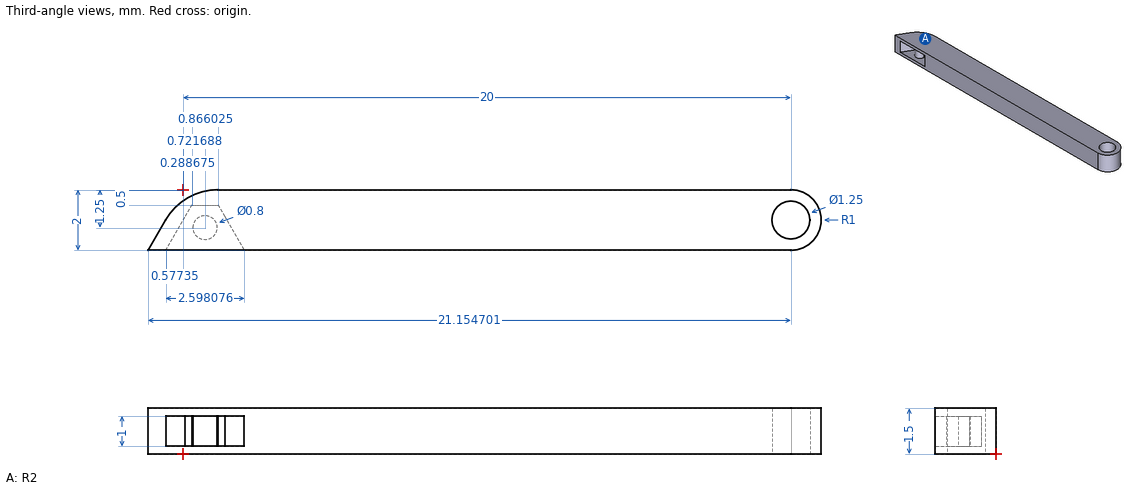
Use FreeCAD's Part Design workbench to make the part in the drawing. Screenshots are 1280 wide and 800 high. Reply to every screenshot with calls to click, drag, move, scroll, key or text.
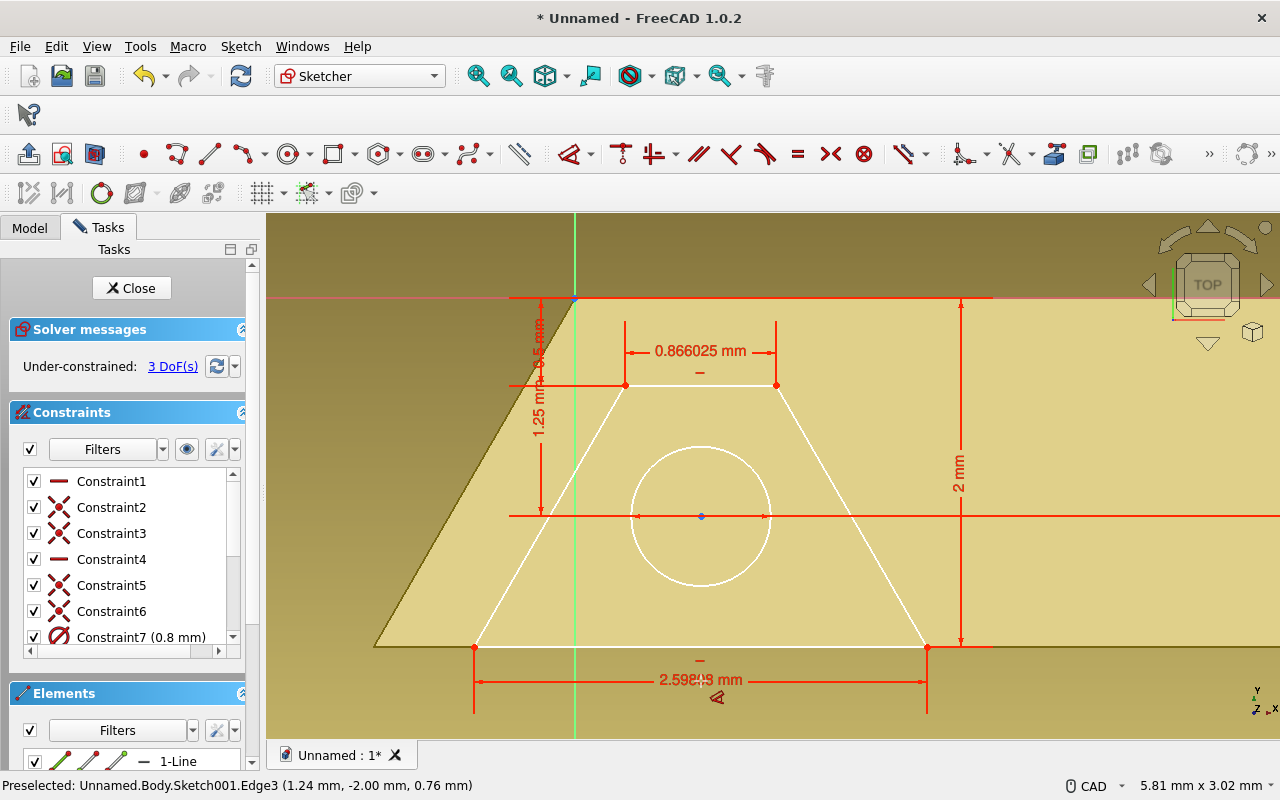
click(474, 647)
click(524, 681)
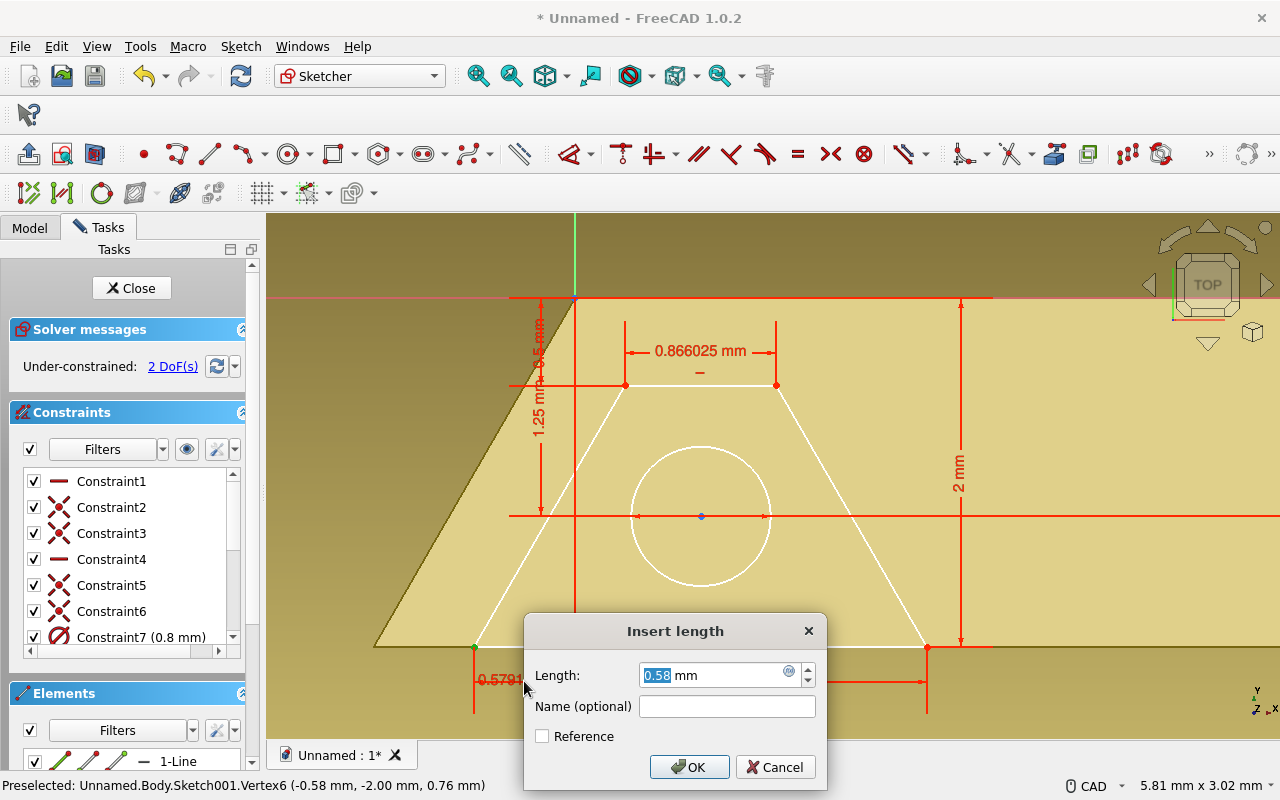
text(0.57735)
key(Return)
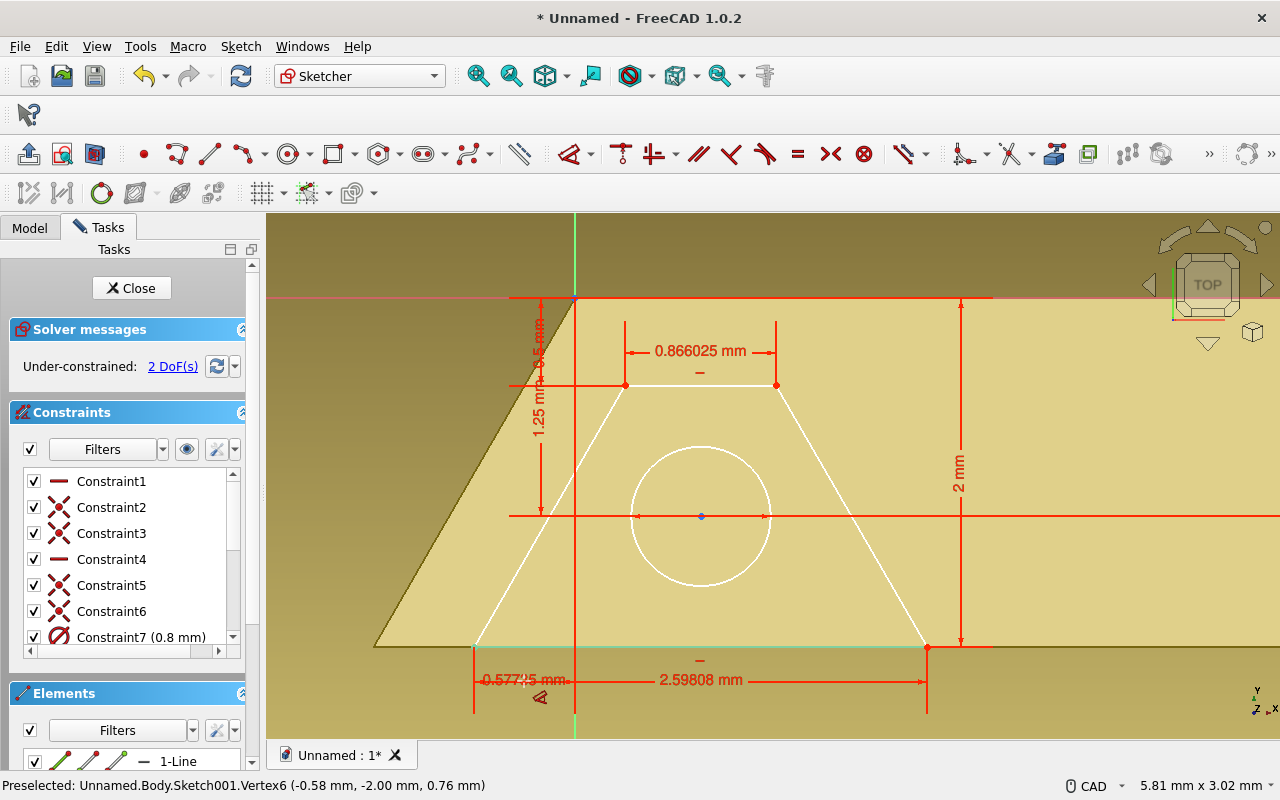
click(701, 516)
click(638, 264)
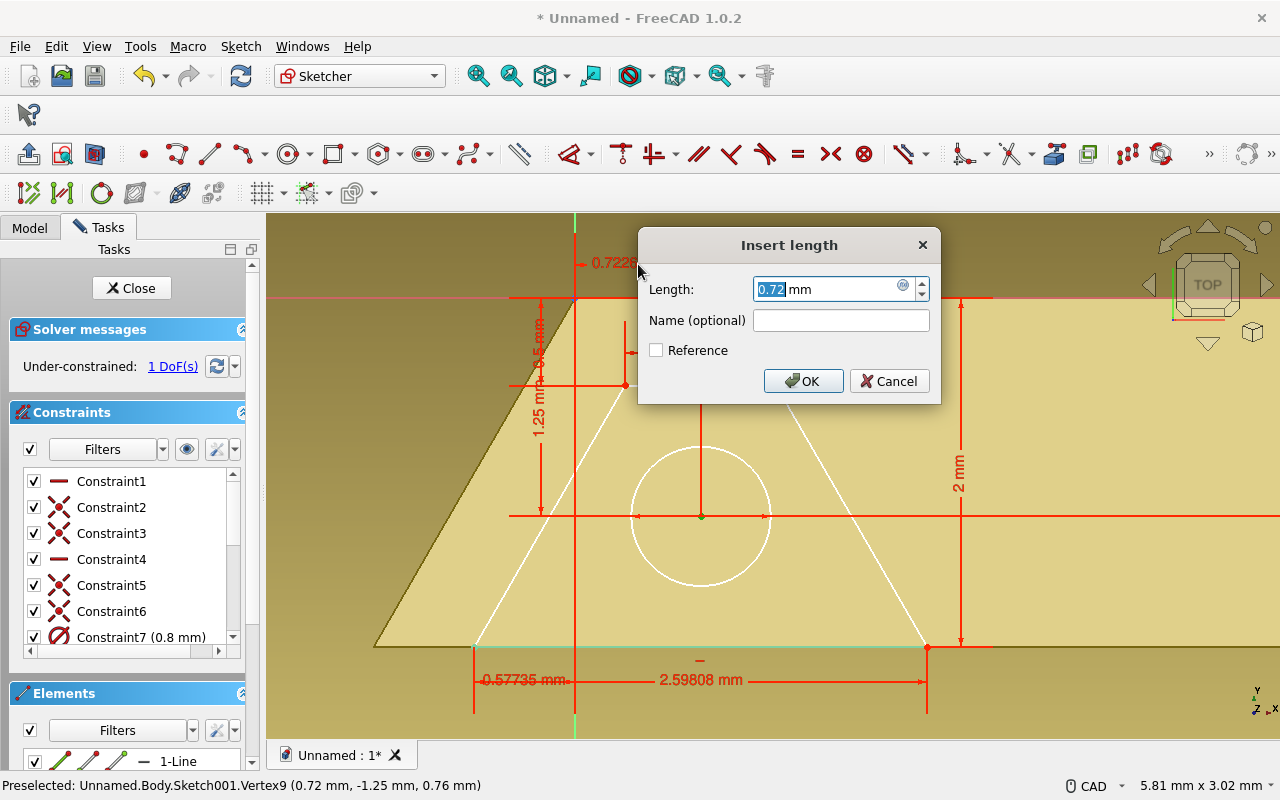
text(0.721688)
key(Return)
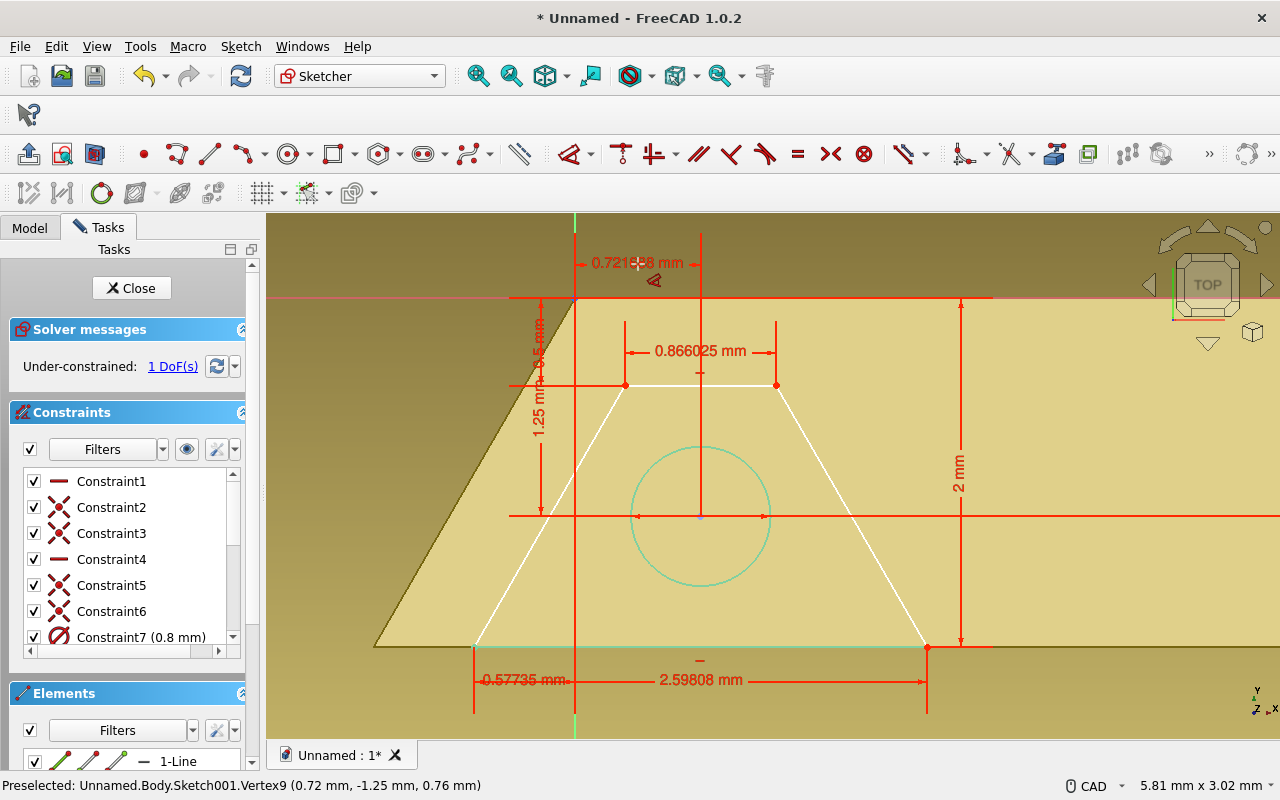
click(625, 386)
click(611, 444)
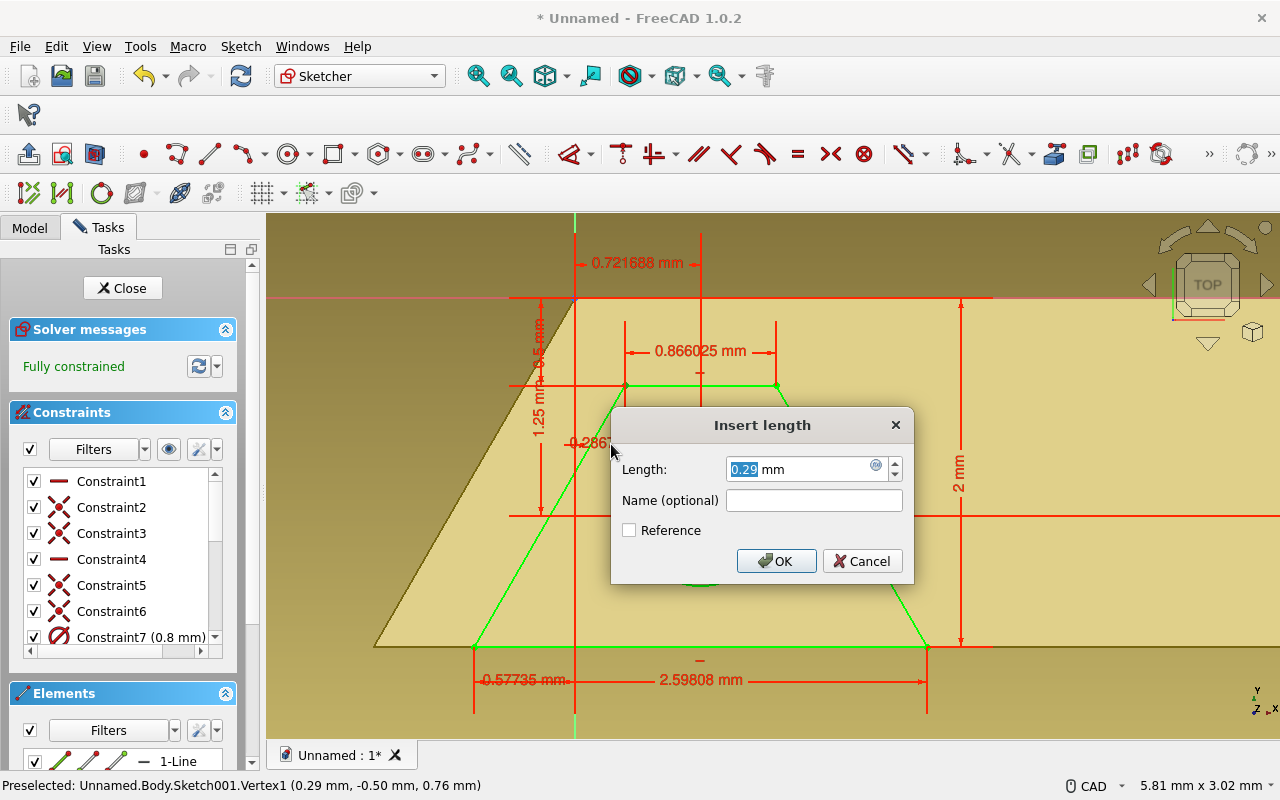
text(0.288675)
key(Return)
key(Escape)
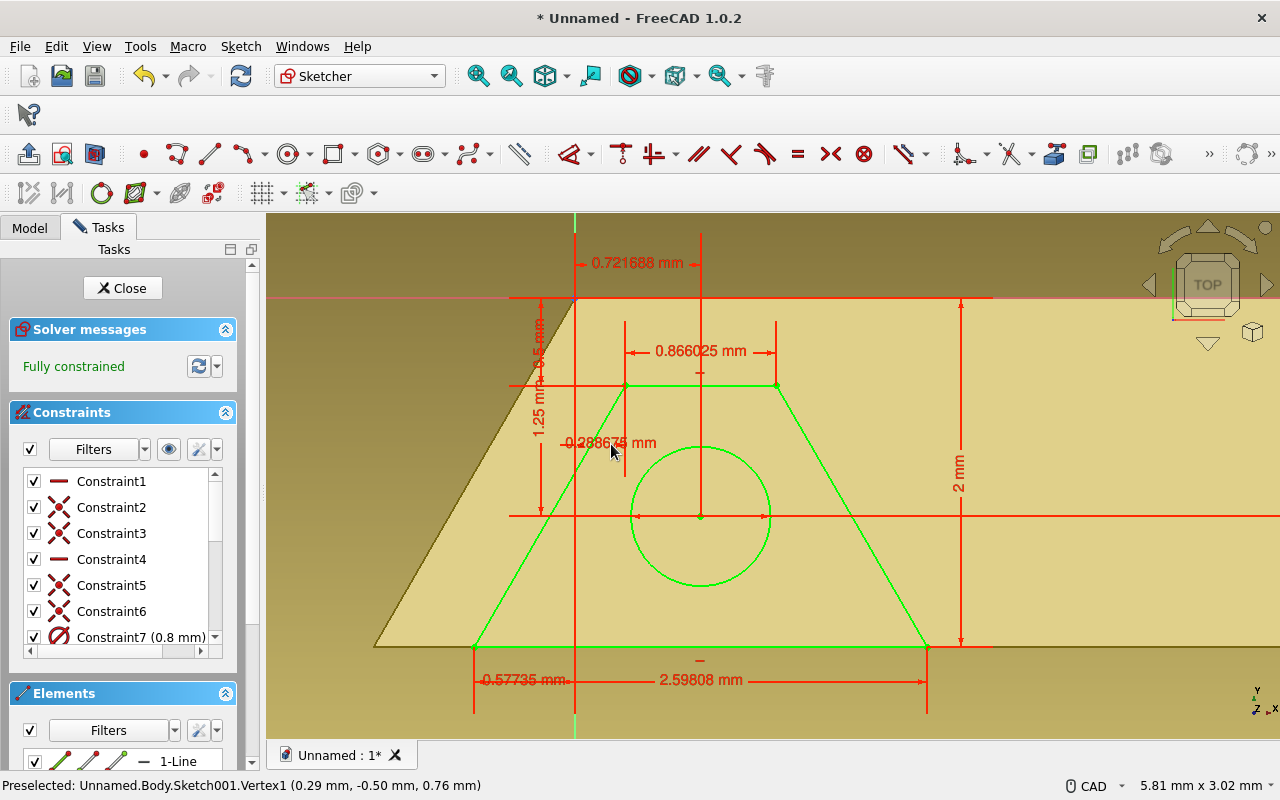
click(123, 288)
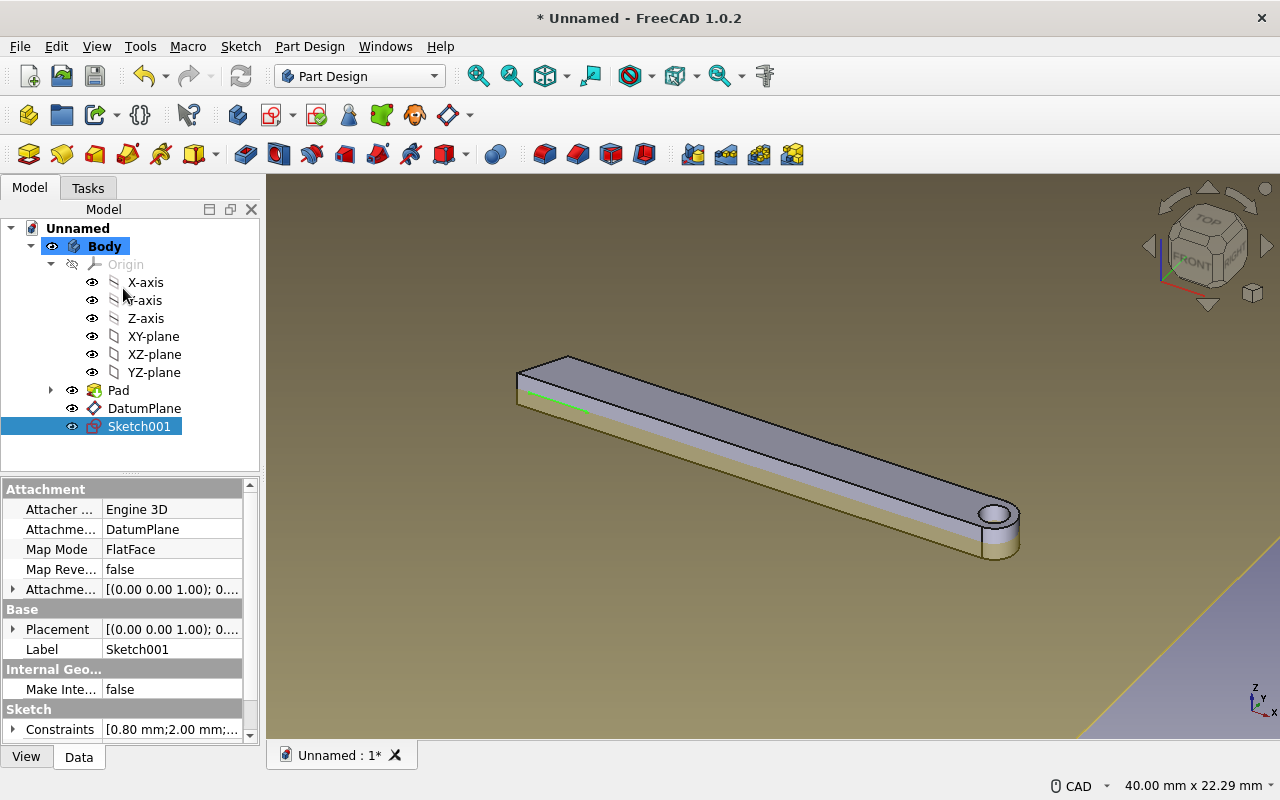
click(246, 154)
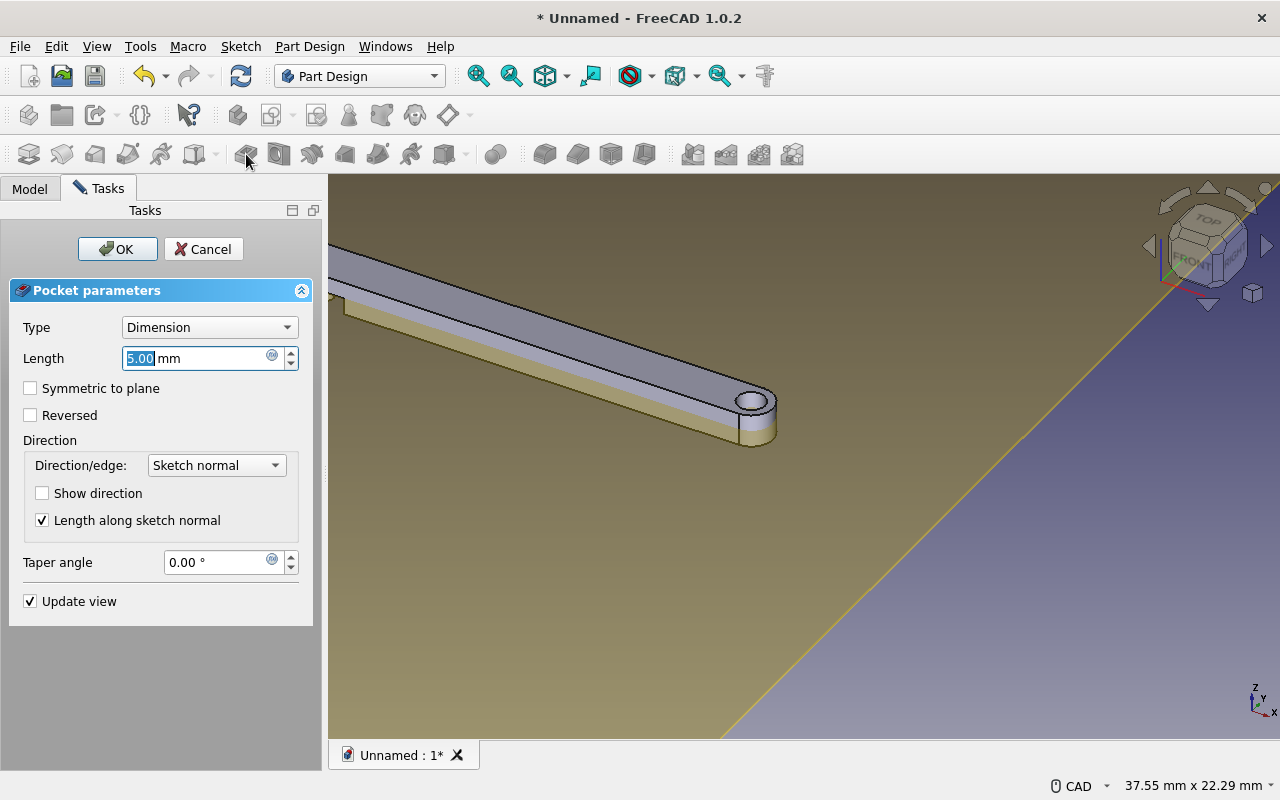
text(1)
key(Tab)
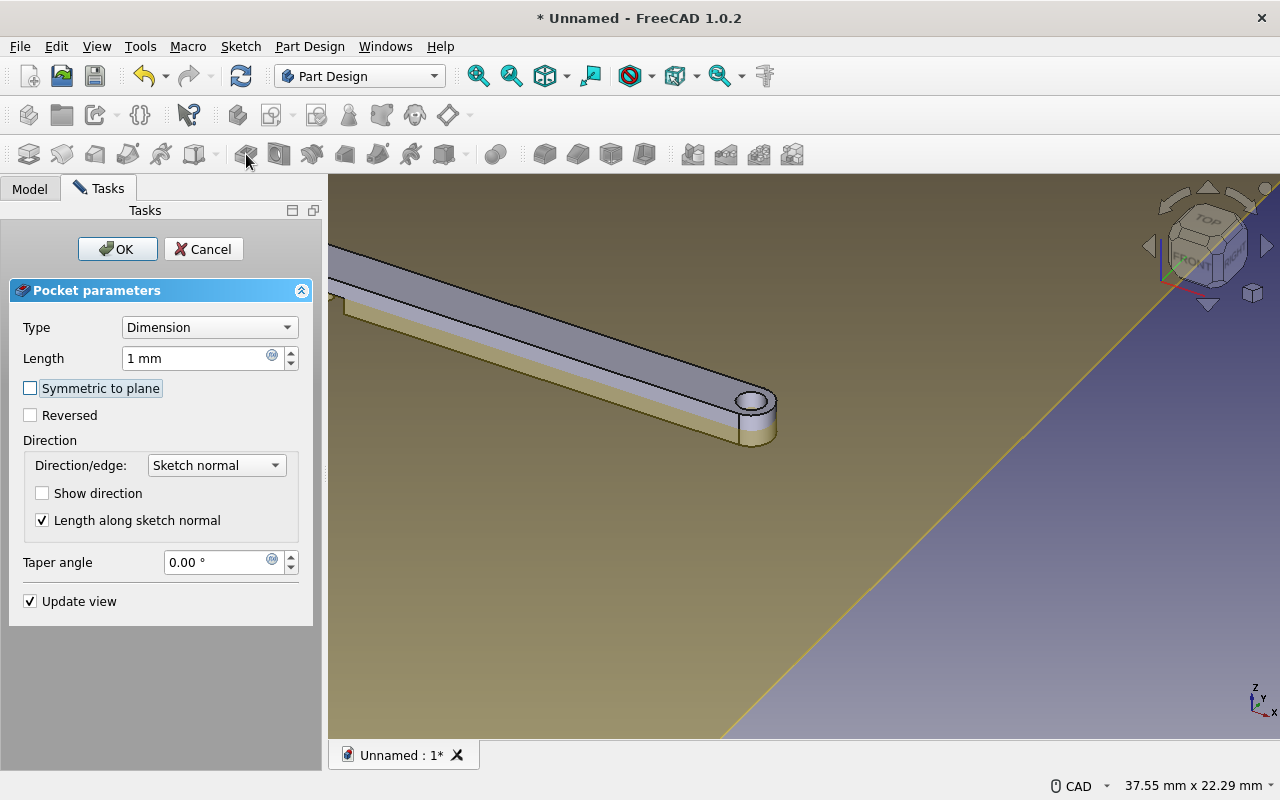
click(31, 388)